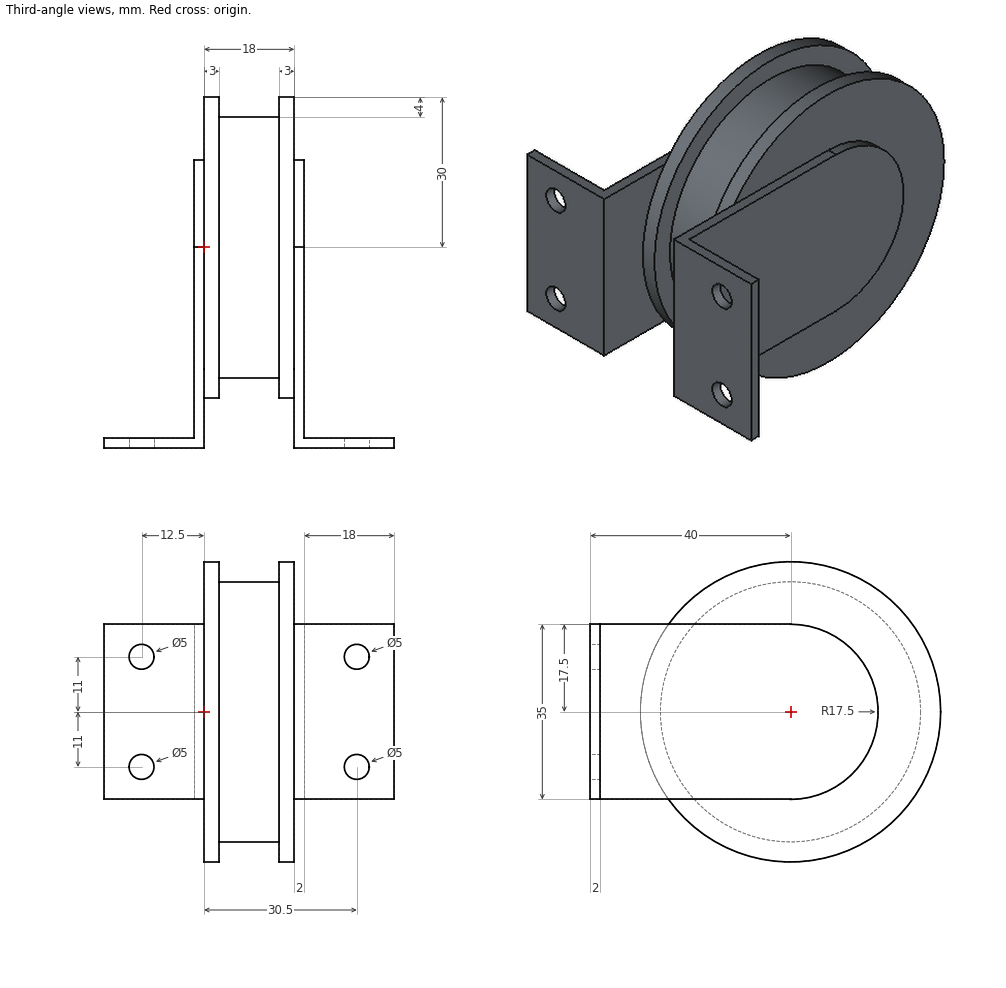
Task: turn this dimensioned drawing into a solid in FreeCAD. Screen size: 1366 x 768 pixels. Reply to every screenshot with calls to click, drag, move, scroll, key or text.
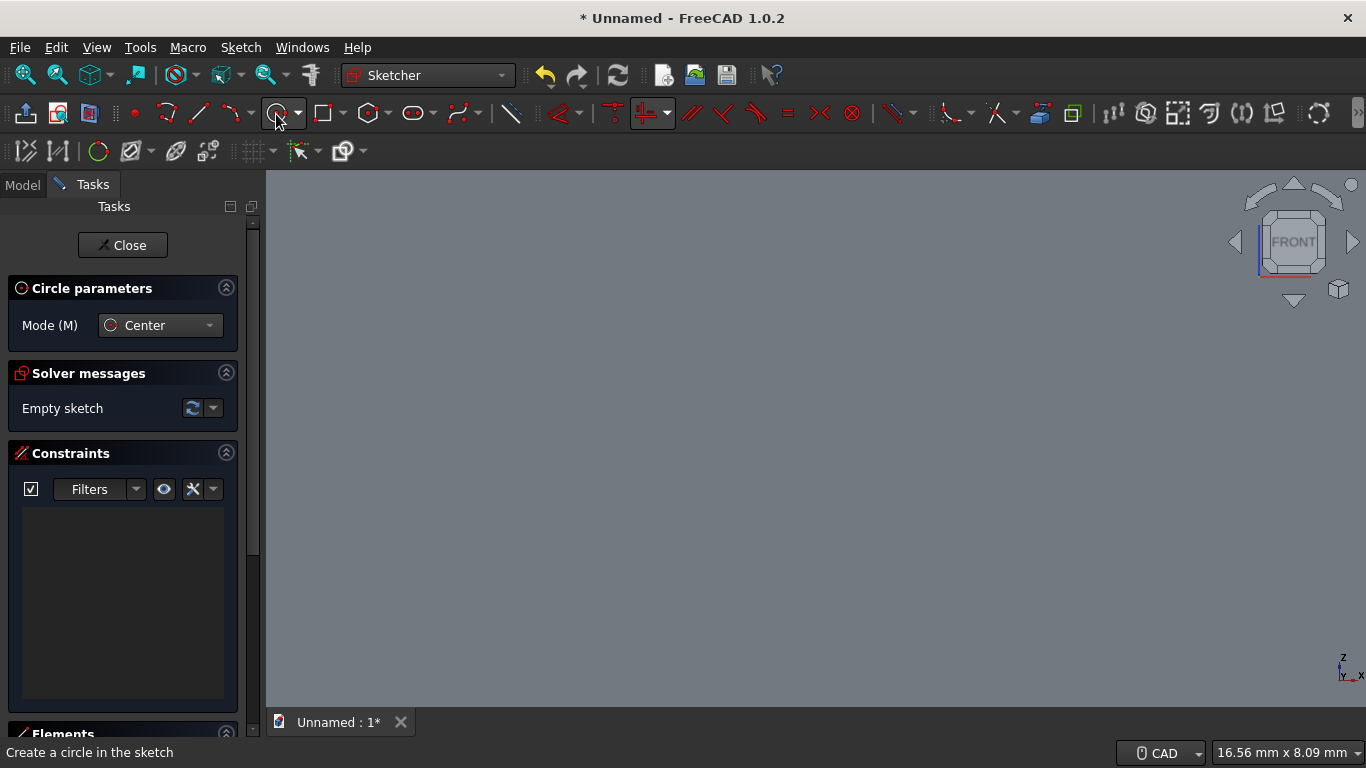
click(742, 432)
click(859, 315)
key(Escape)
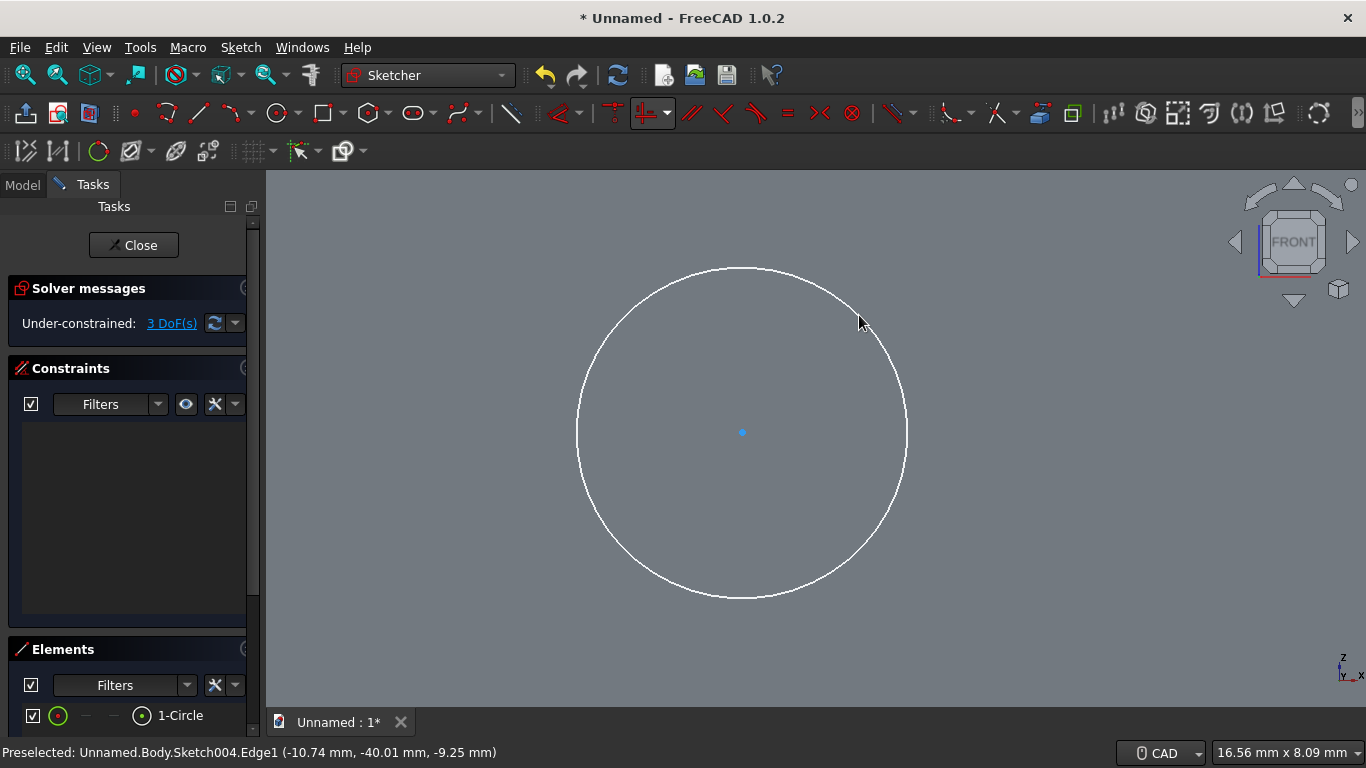
click(558, 114)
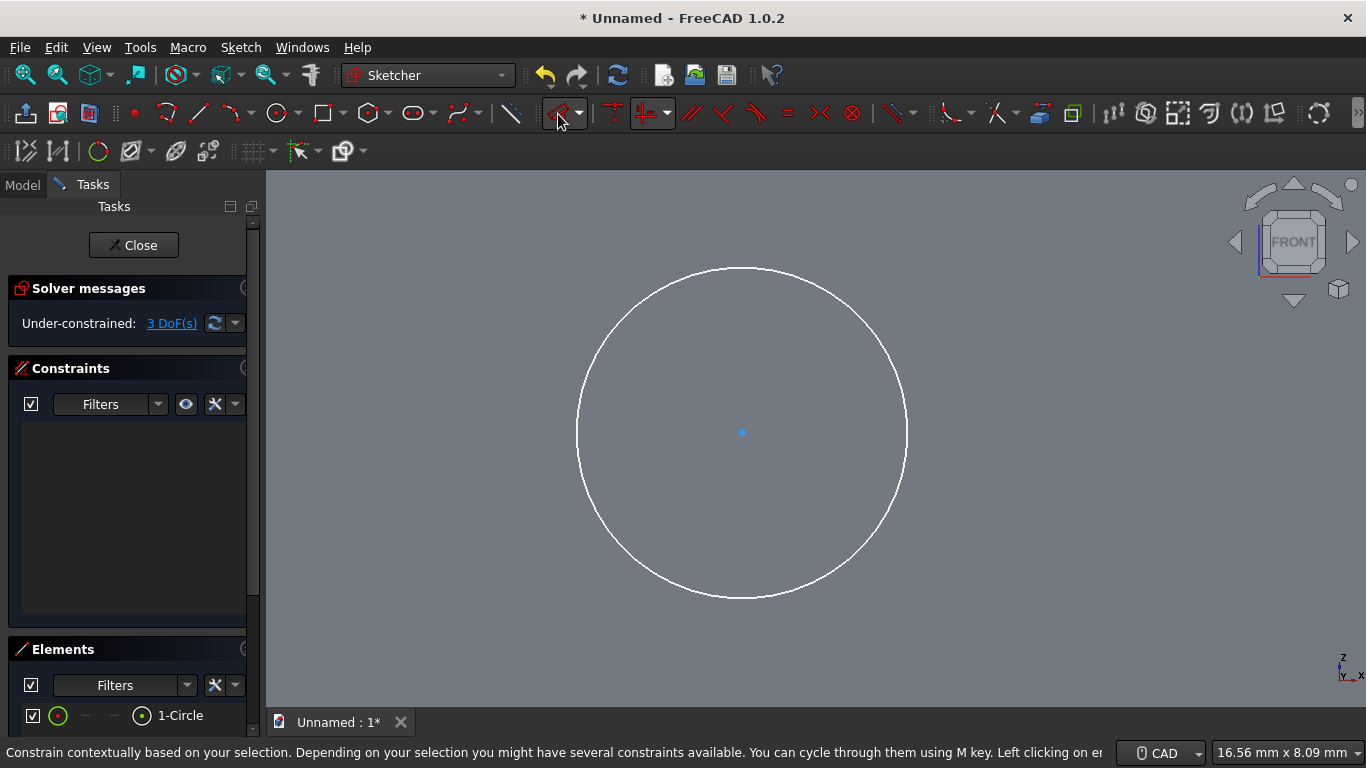
click(859, 316)
click(882, 293)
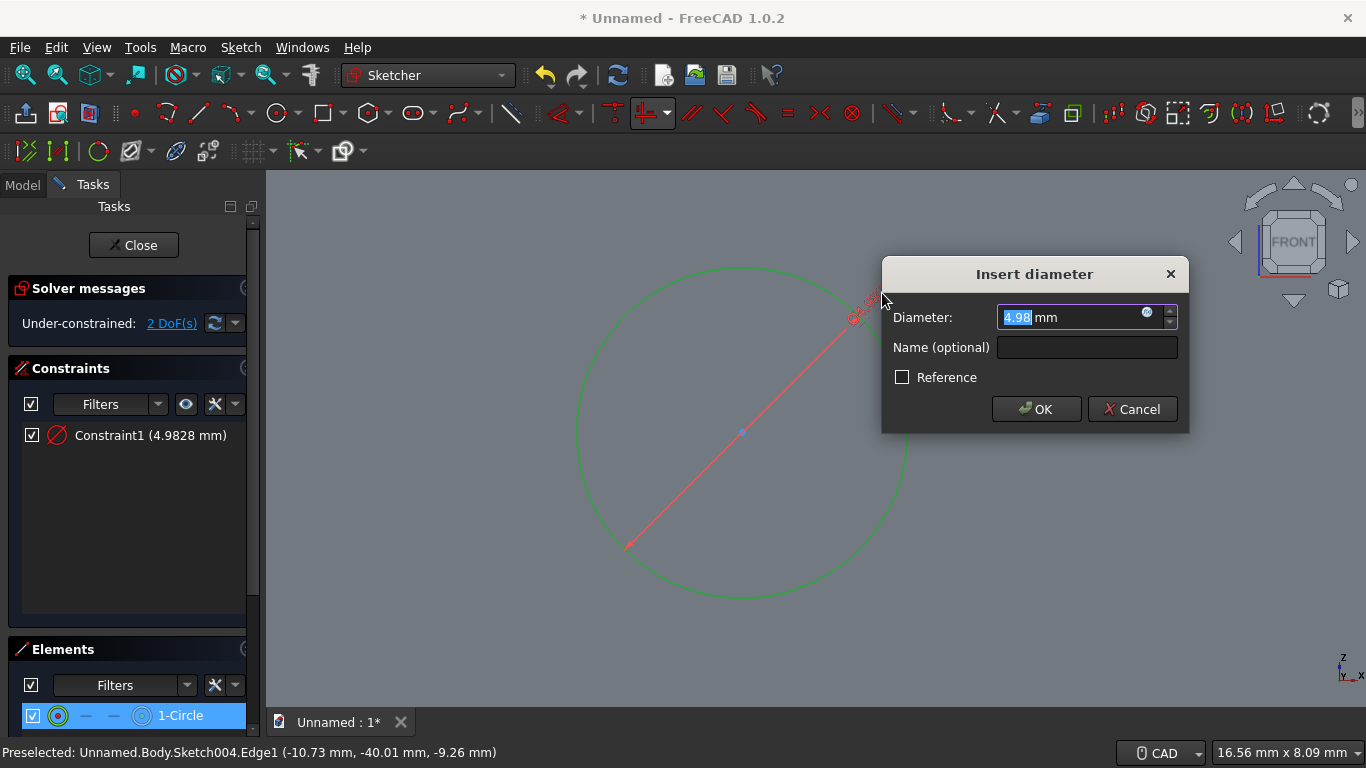
text(5)
key(Return)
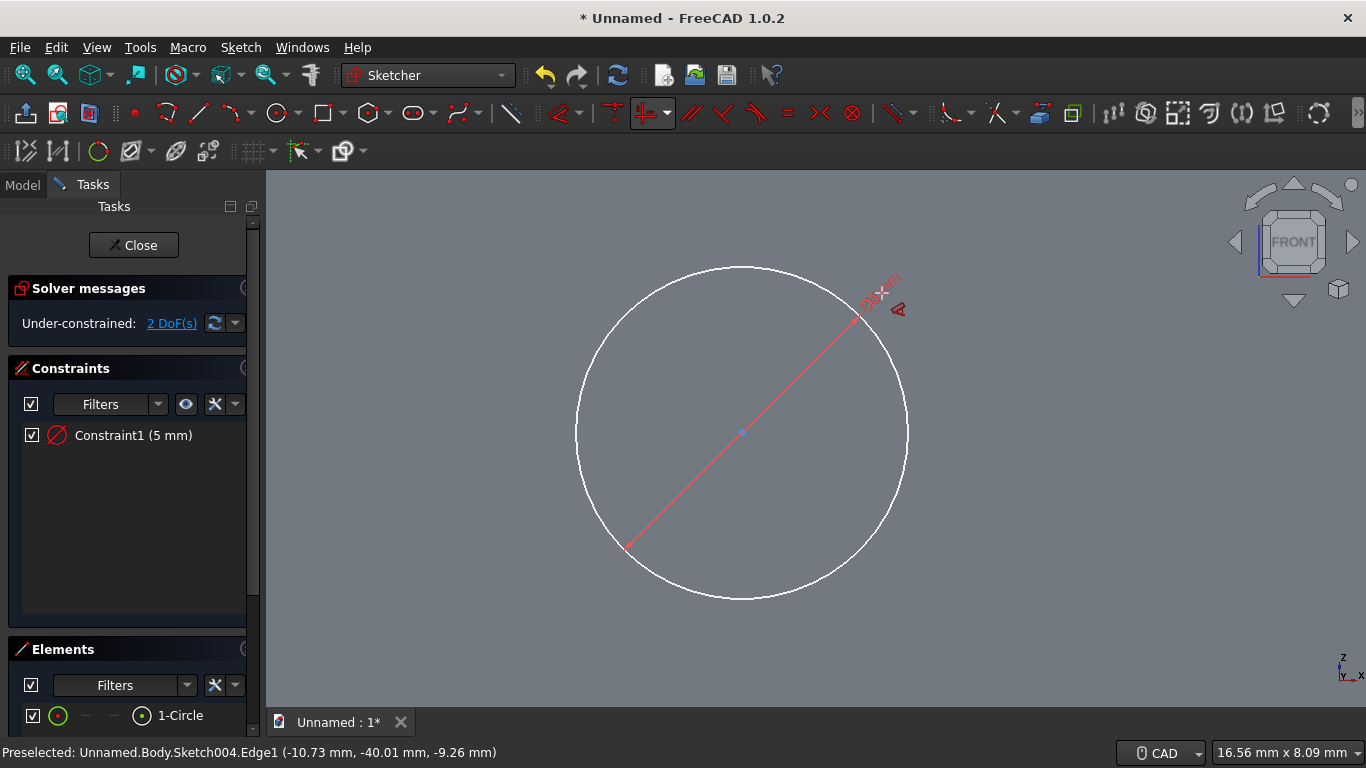
click(742, 433)
click(708, 315)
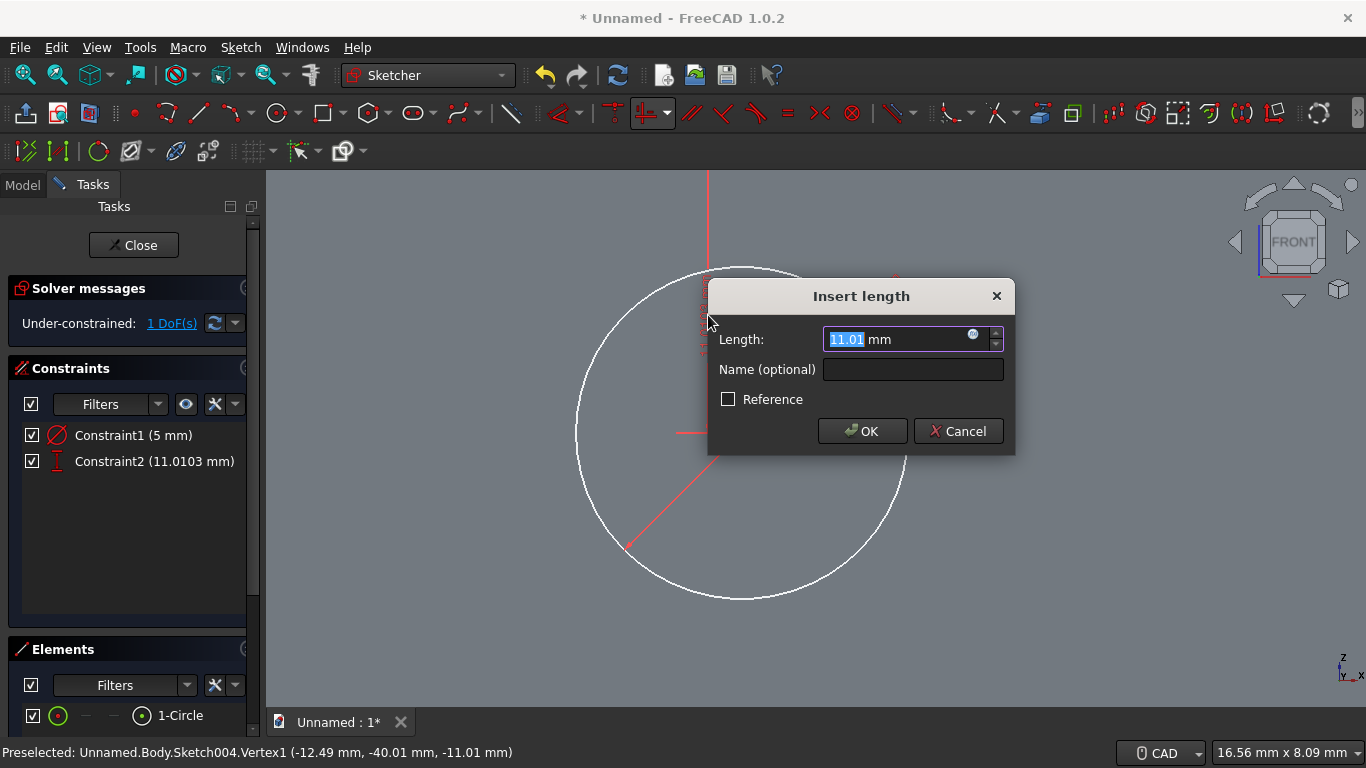
text(11)
key(Return)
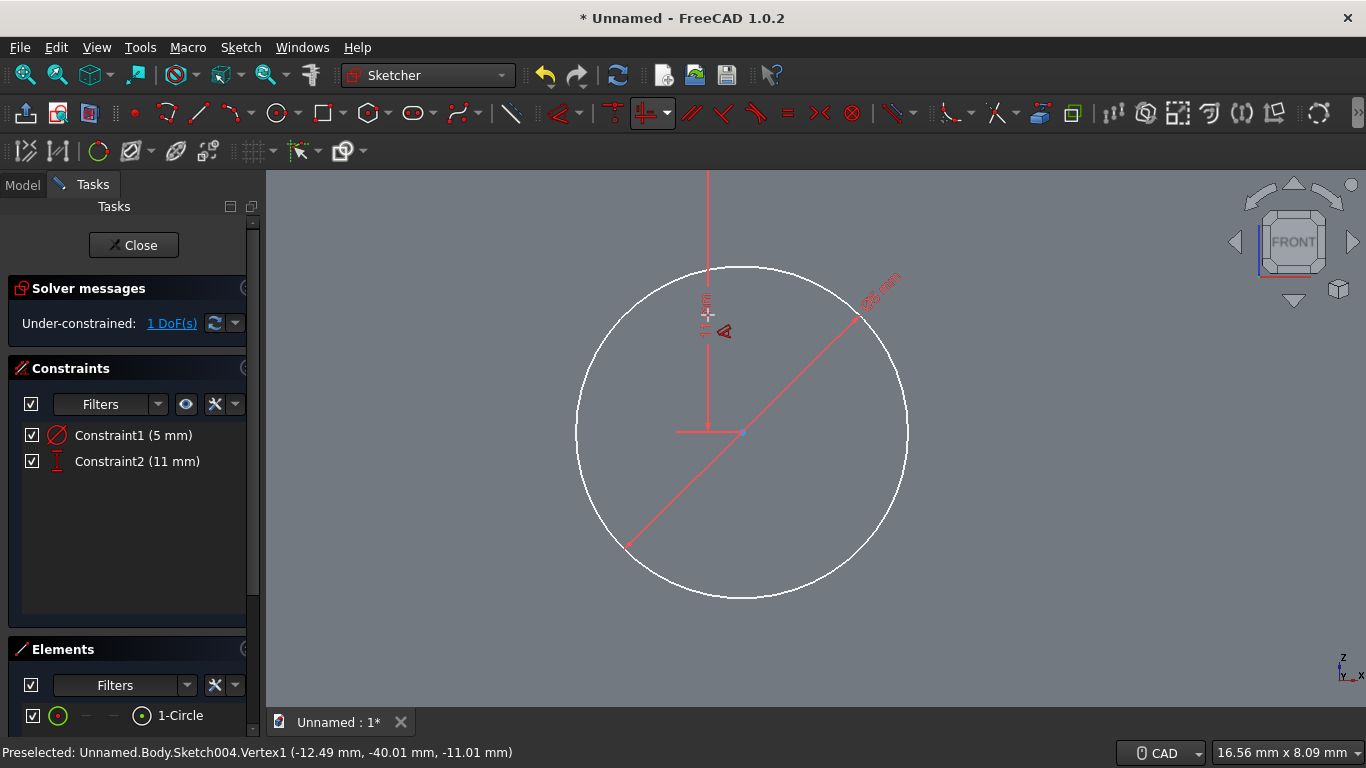
click(742, 432)
click(971, 466)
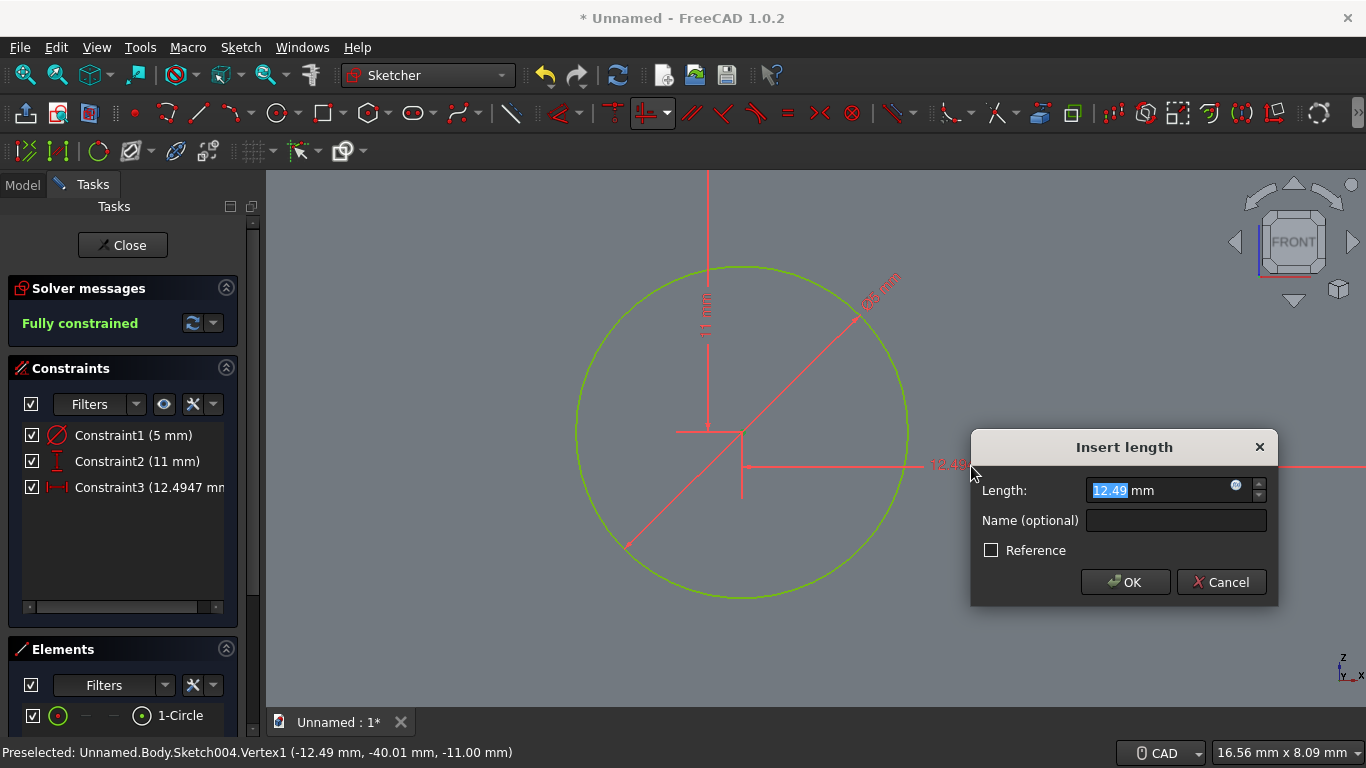
text(12.5)
key(Return)
key(Escape)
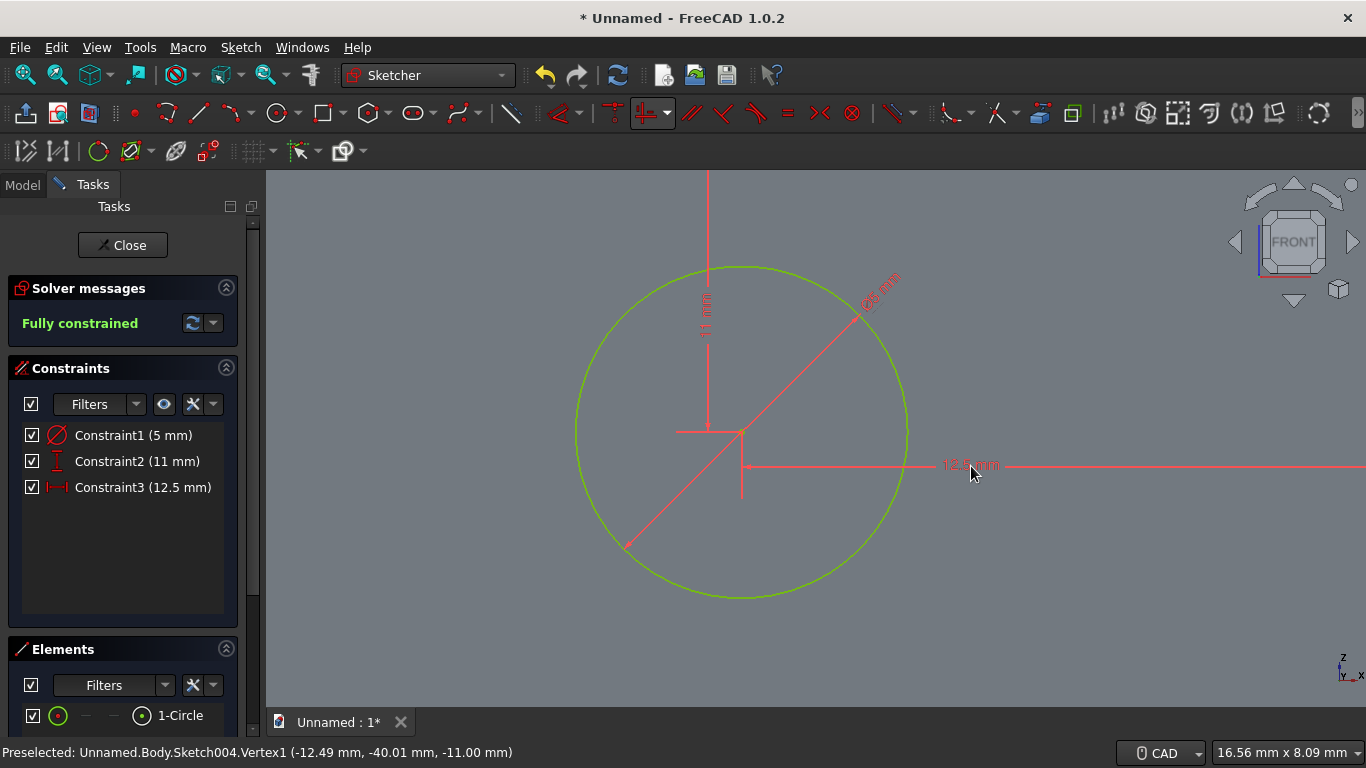
click(123, 245)